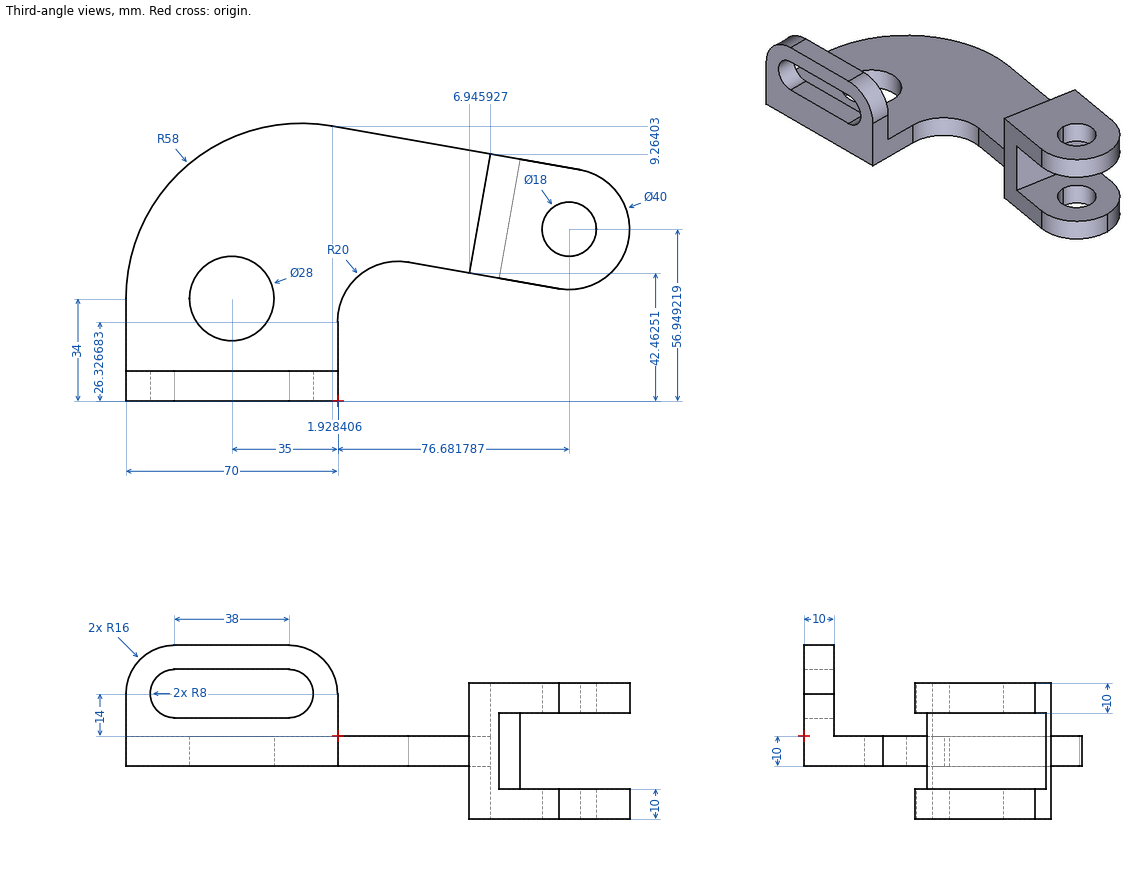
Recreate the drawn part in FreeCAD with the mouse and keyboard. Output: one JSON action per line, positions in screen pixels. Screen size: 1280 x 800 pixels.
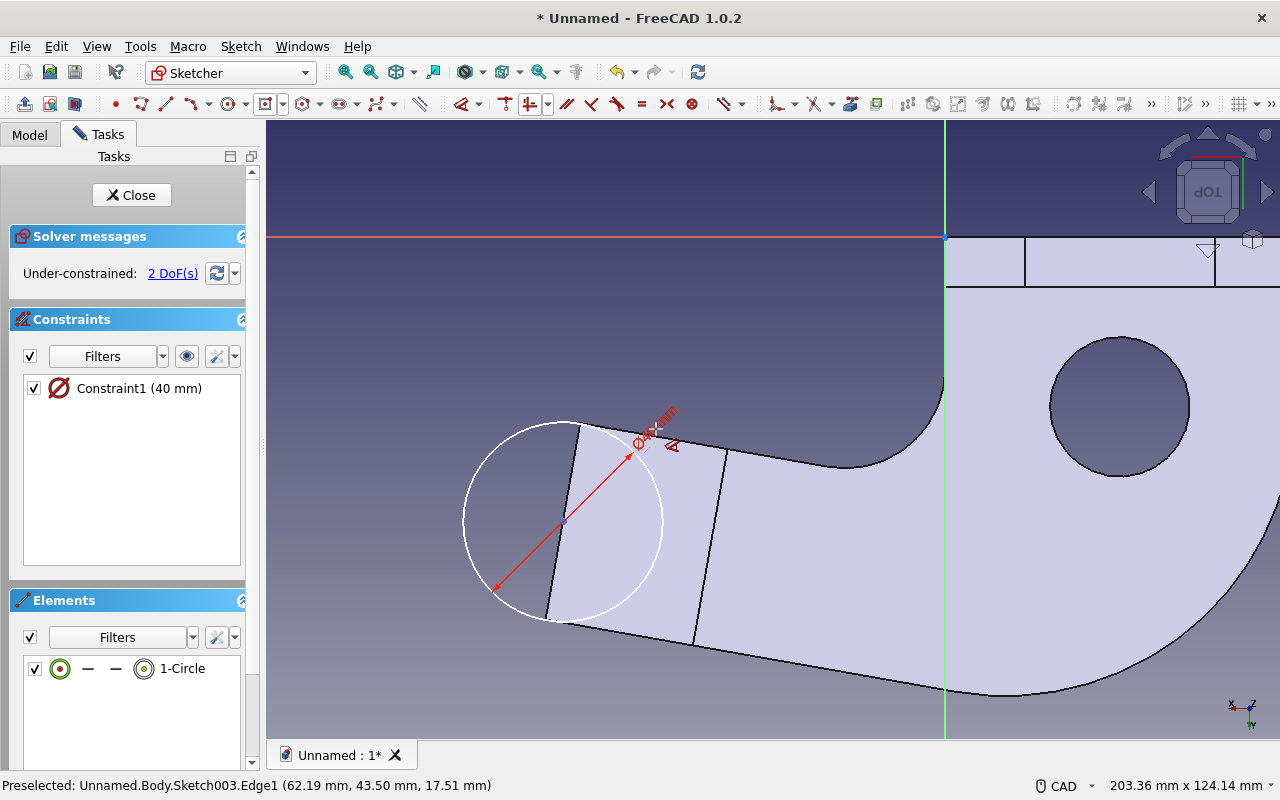
{"action": "left_click", "coordinate": [563, 522]}
{"action": "left_click", "coordinate": [754, 203]}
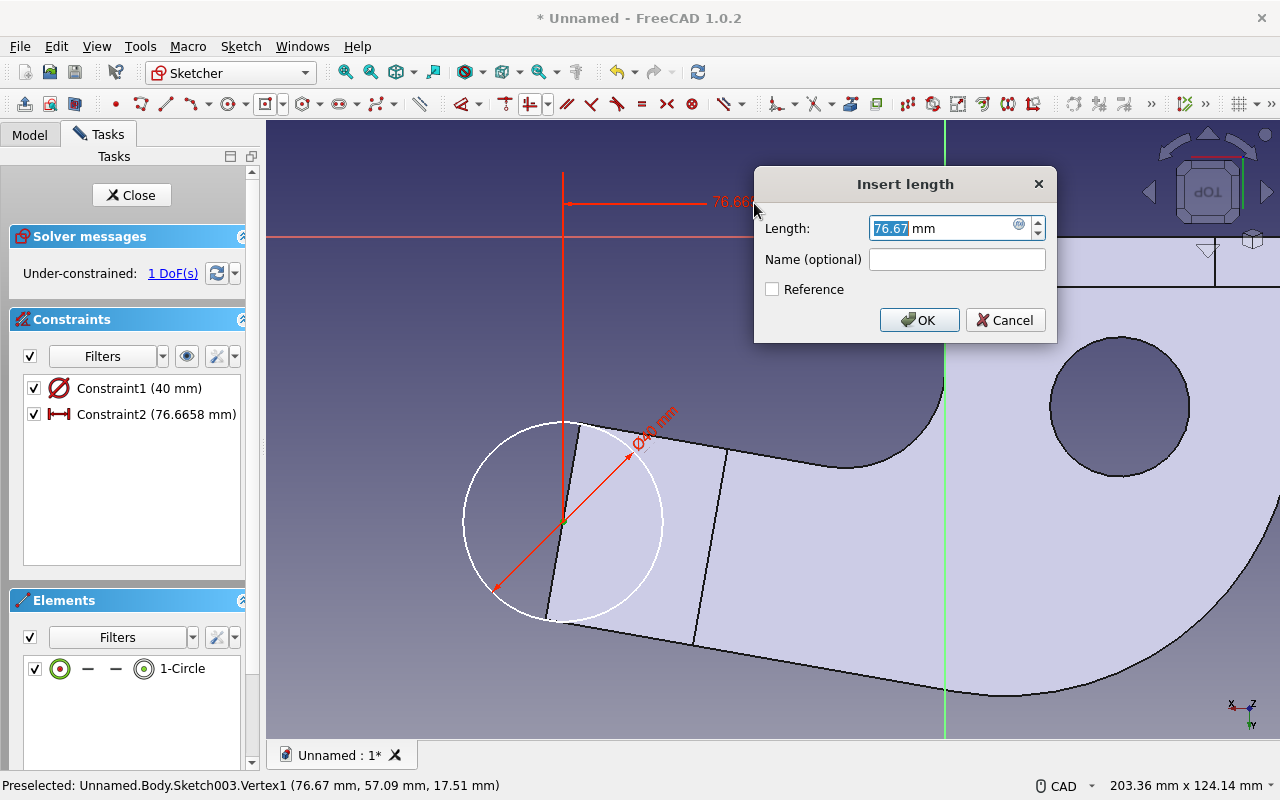
{"action": "type", "text": "76.681787"}
{"action": "key", "text": "Return"}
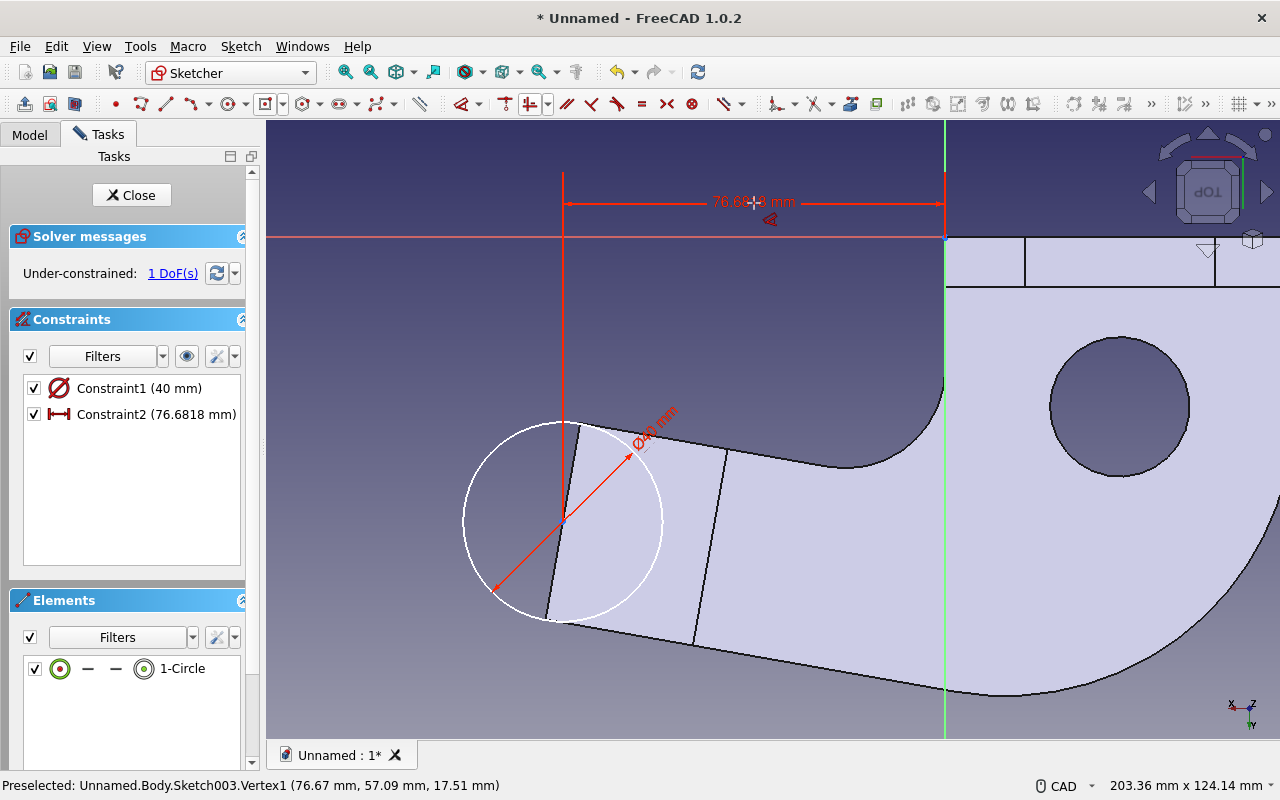
{"action": "left_click", "coordinate": [563, 522]}
{"action": "left_click", "coordinate": [979, 380]}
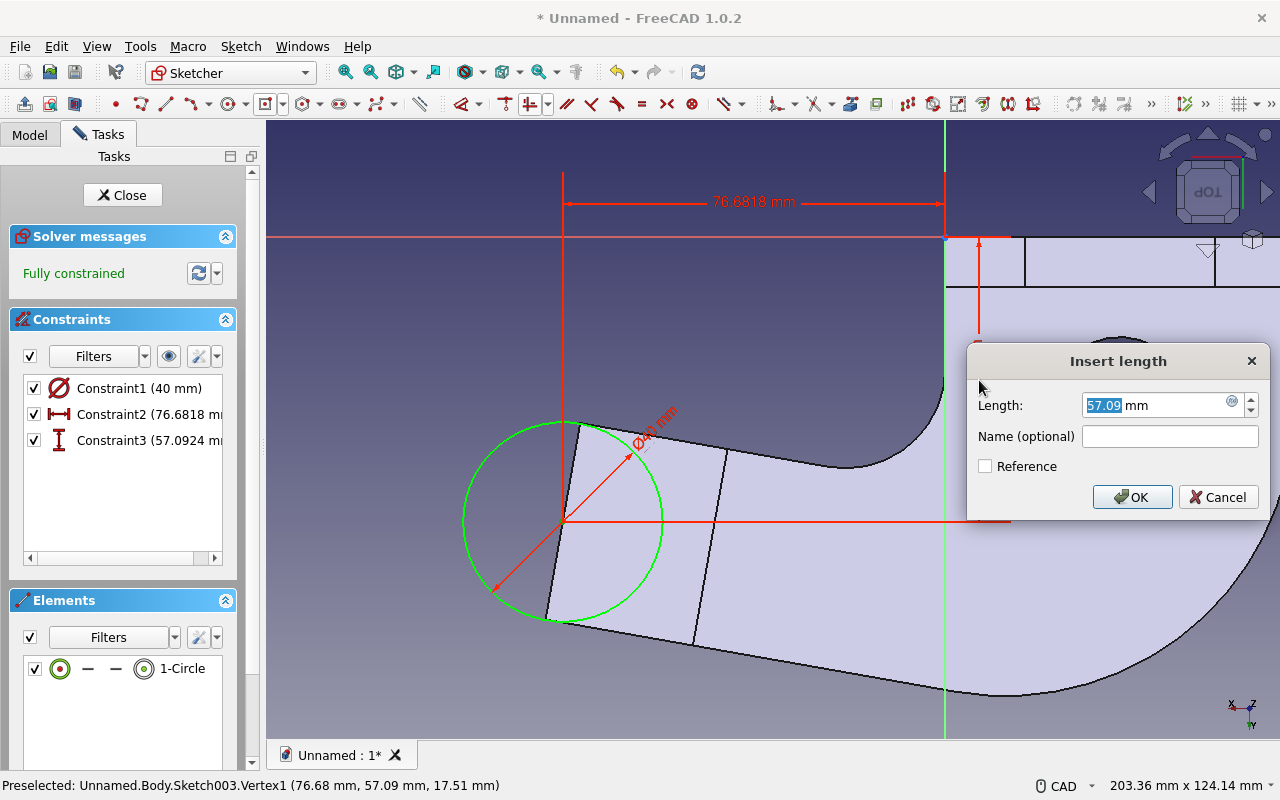
{"action": "type", "text": "56.949219"}
{"action": "key", "text": "Return"}
{"action": "key", "text": "Escape"}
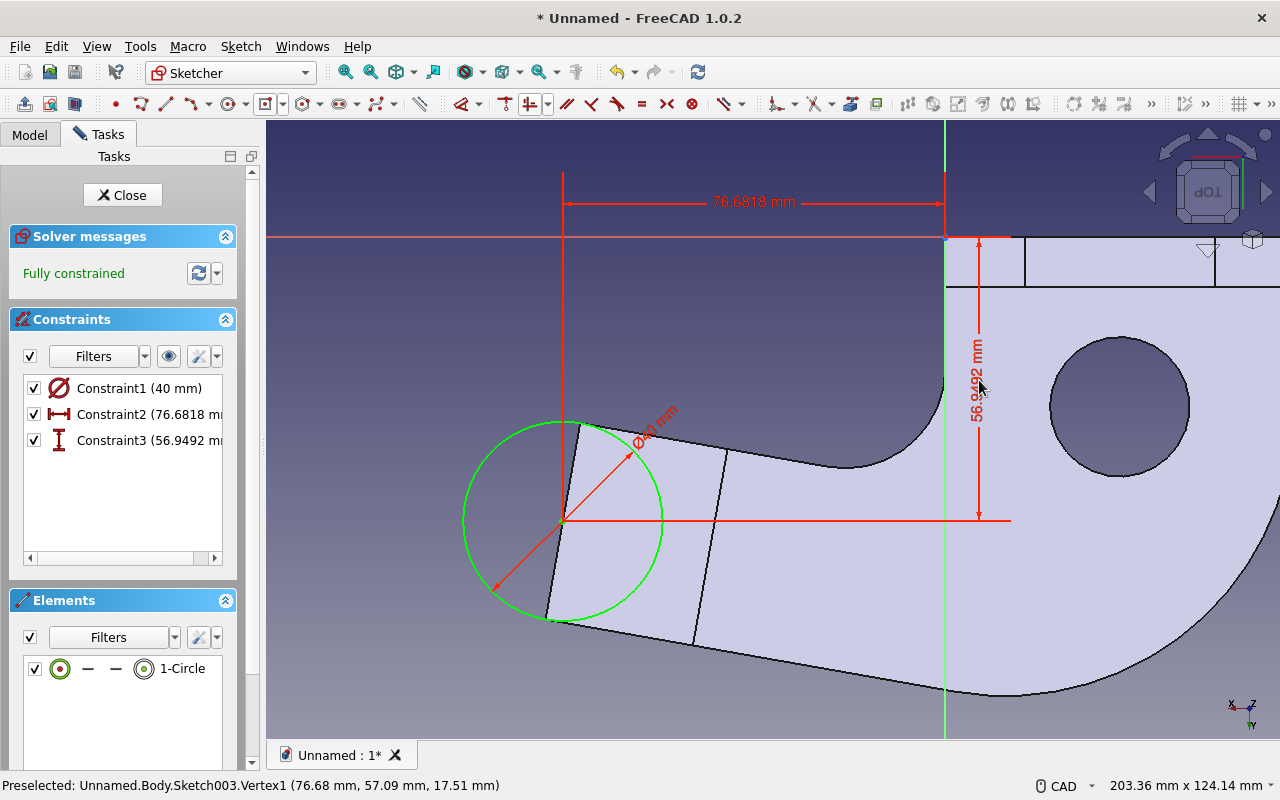
{"action": "left_click", "coordinate": [123, 195]}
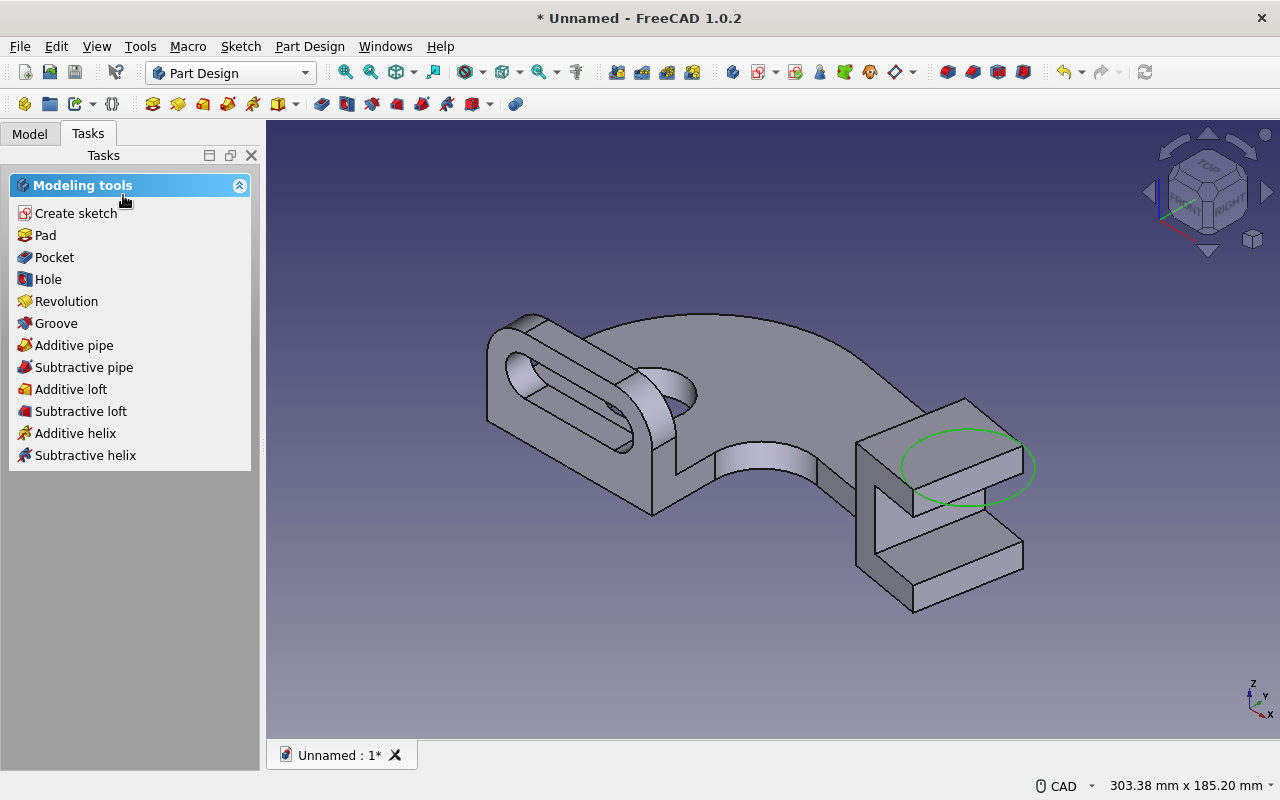
{"action": "left_click", "coordinate": [153, 104]}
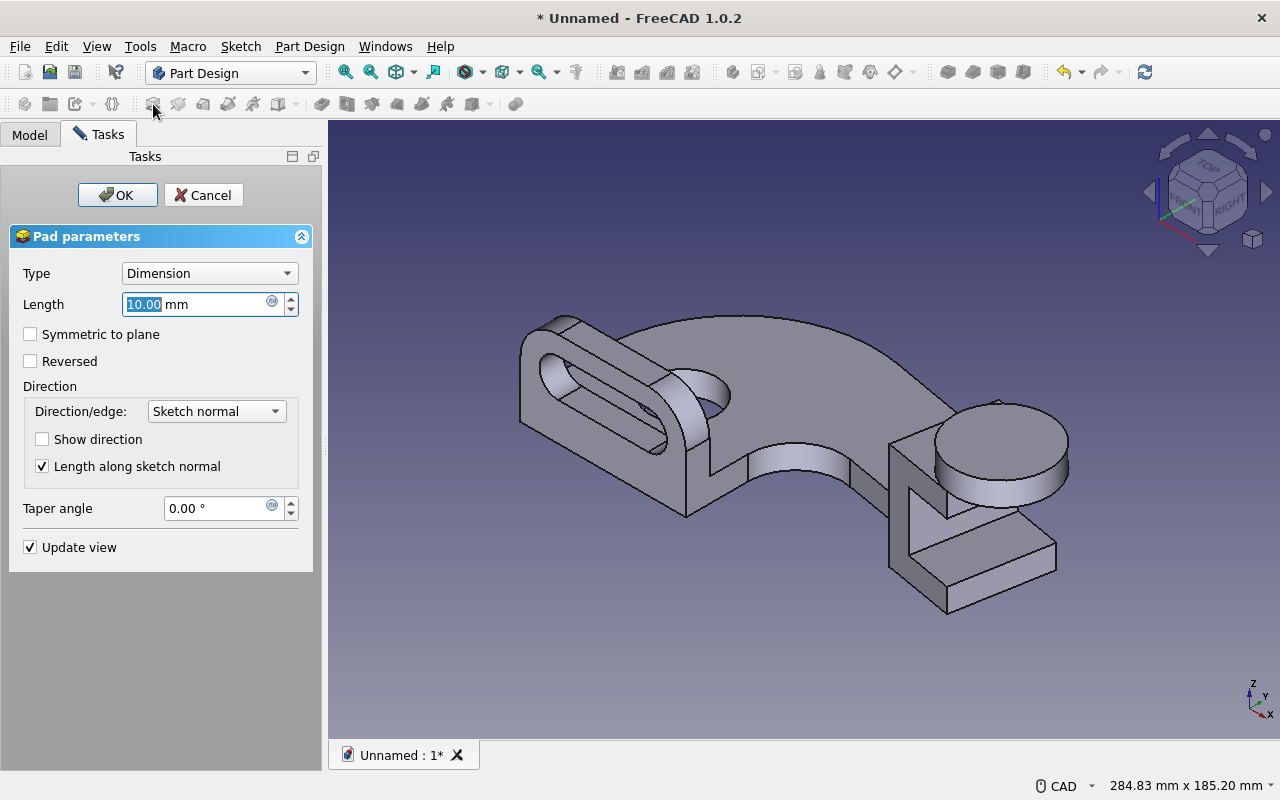
{"action": "type", "text": "10"}
{"action": "key", "text": "Tab"}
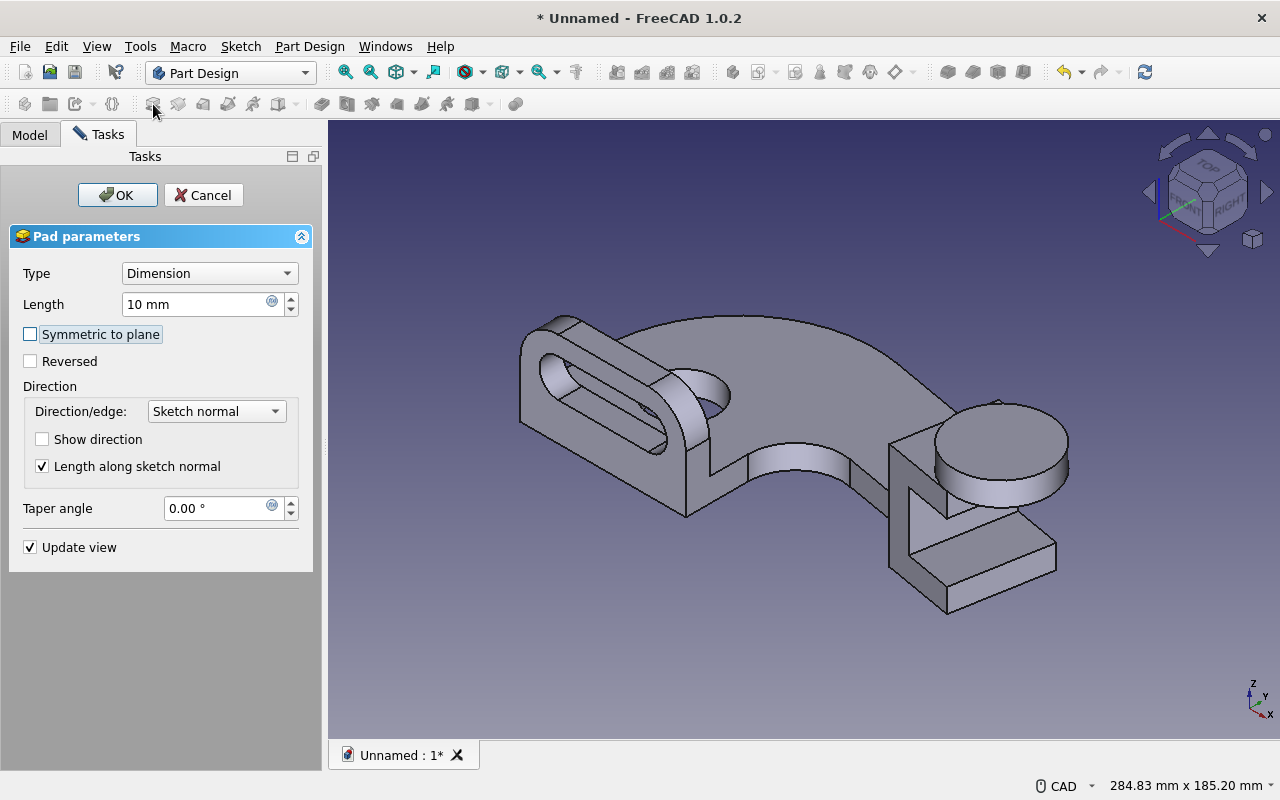
{"action": "left_click", "coordinate": [31, 361]}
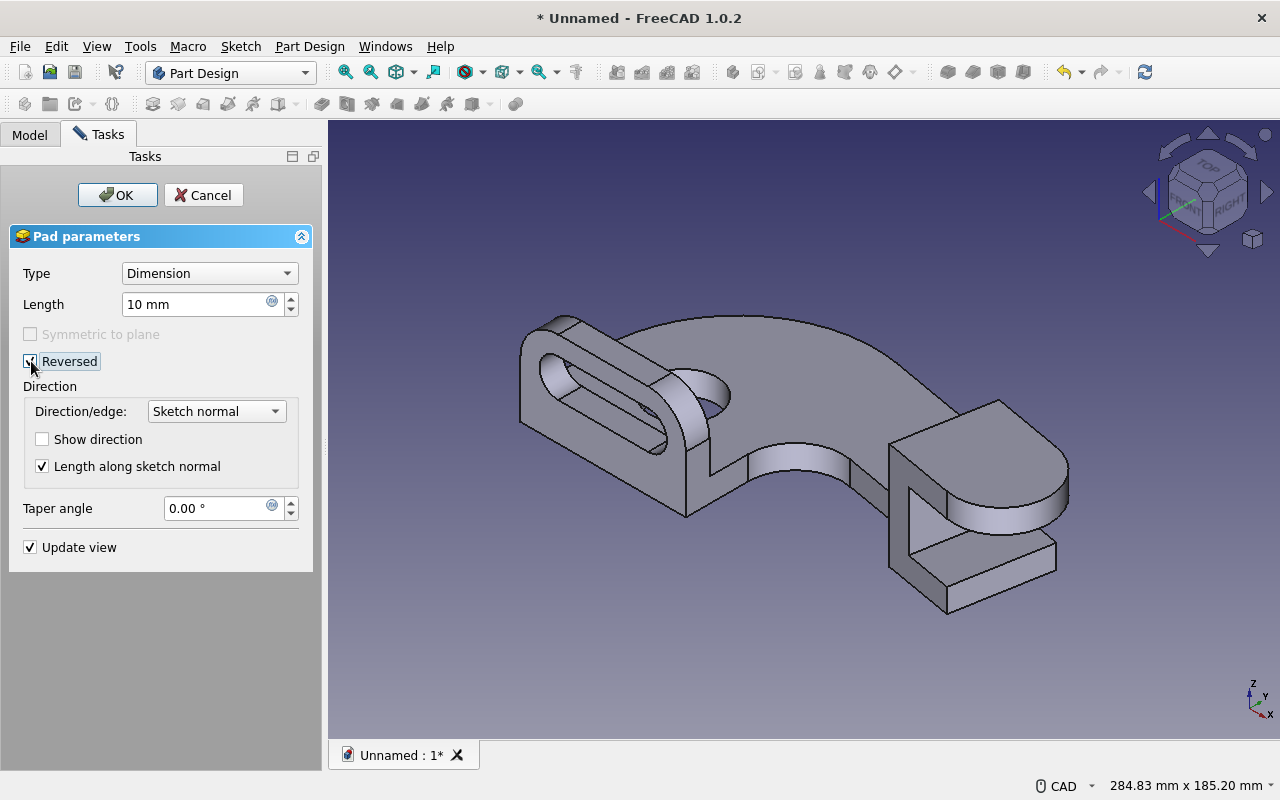
{"action": "left_click", "coordinate": [118, 195]}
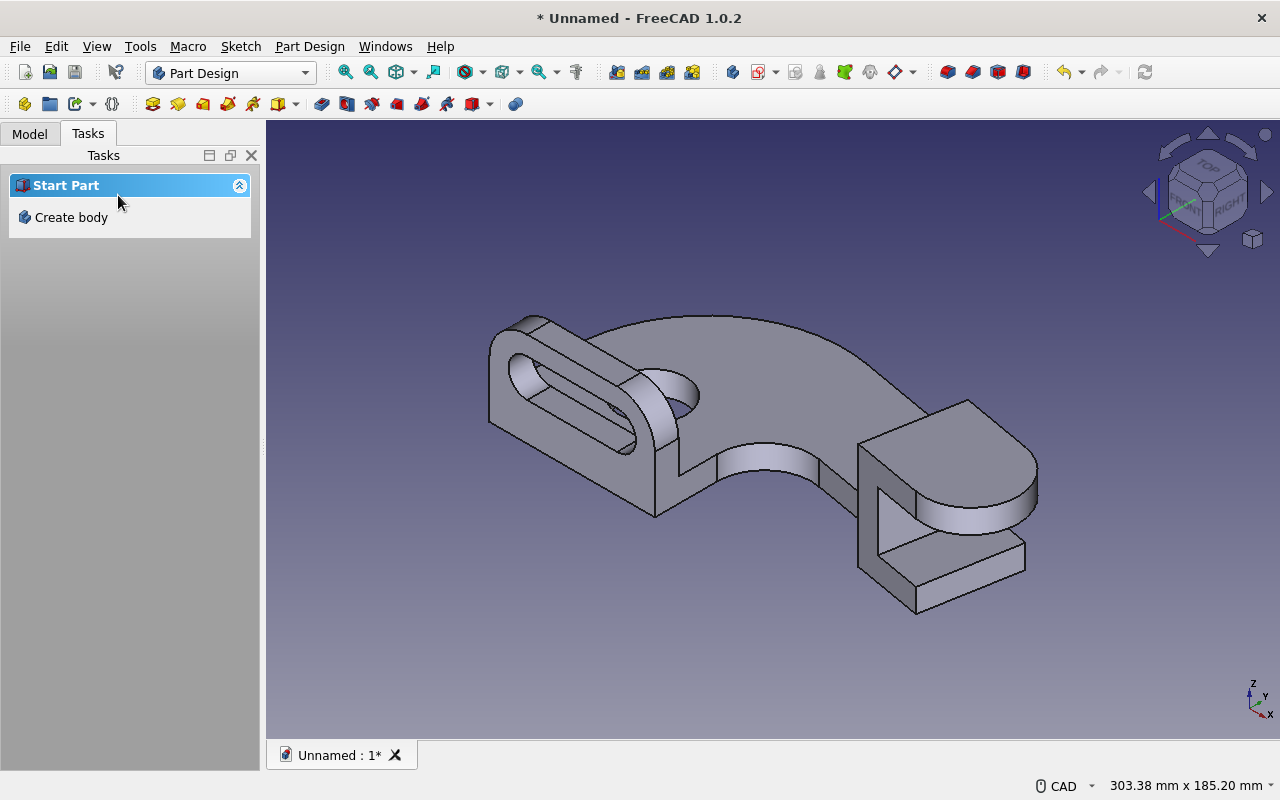
{"action": "left_click", "coordinate": [30, 134]}